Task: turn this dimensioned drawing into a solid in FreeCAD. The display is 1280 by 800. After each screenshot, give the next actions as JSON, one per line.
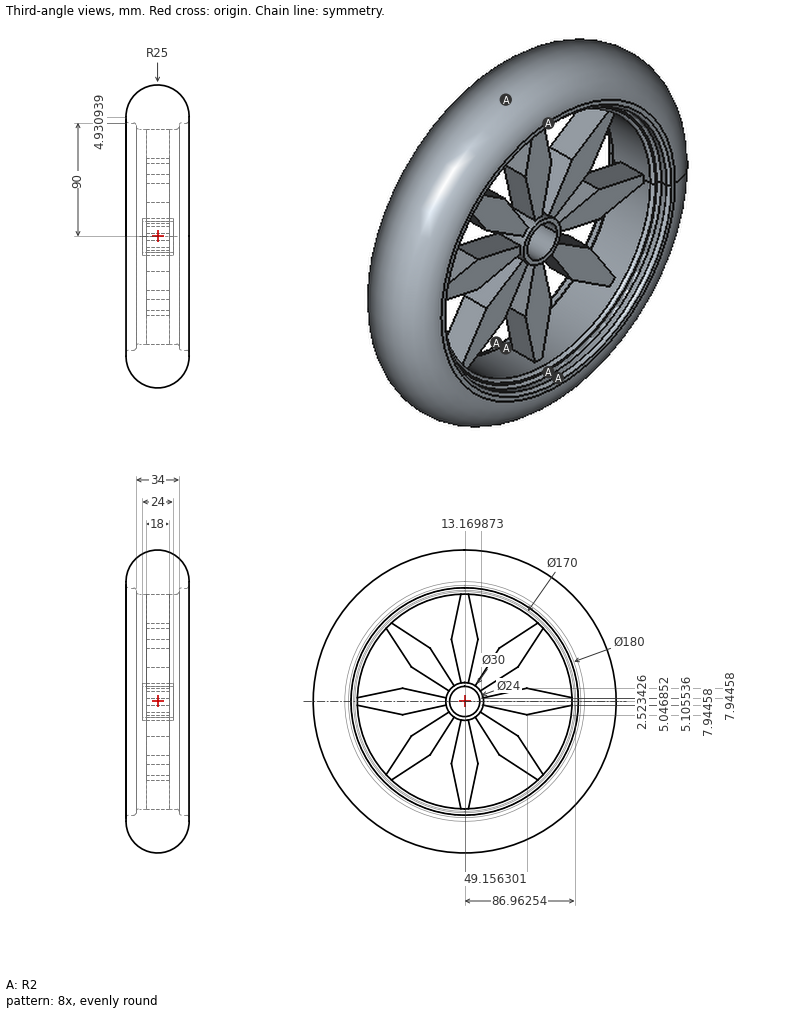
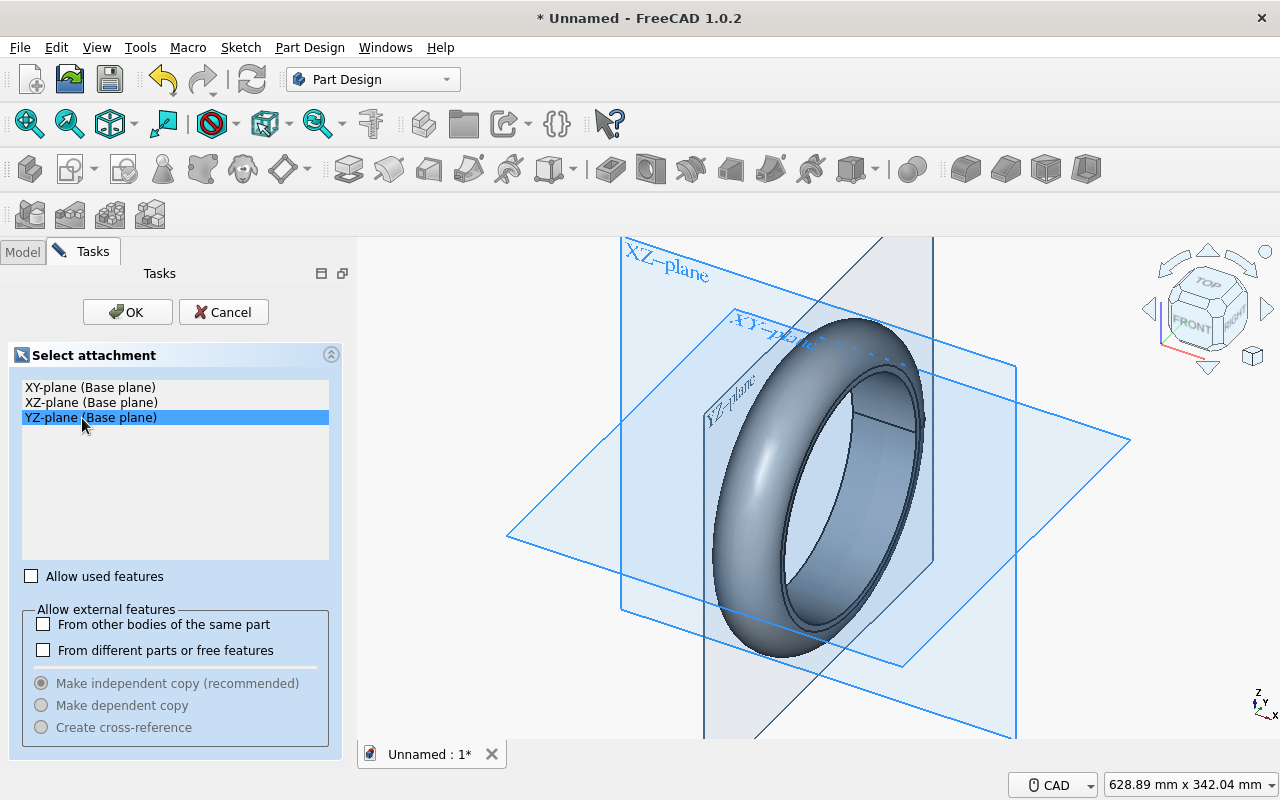
{"action": "left_click", "coordinate": [128, 312]}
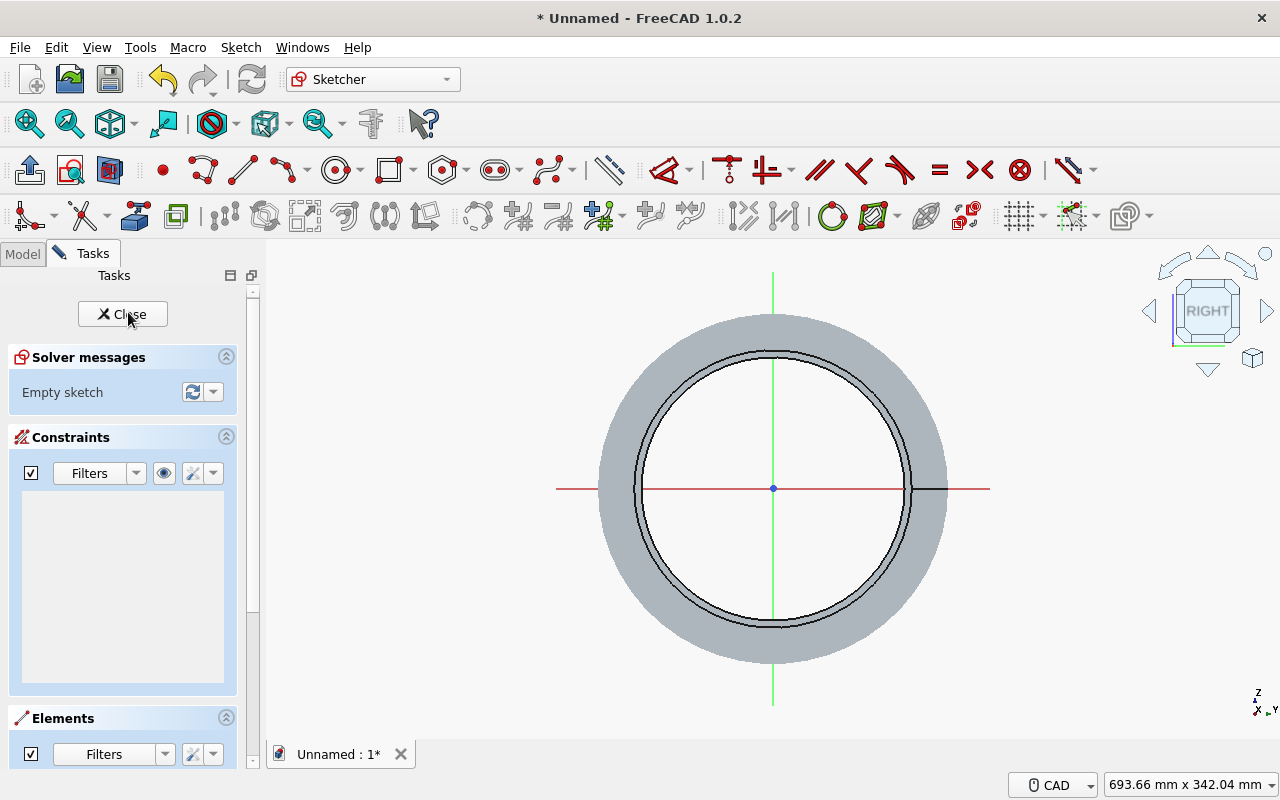
{"action": "left_click", "coordinate": [110, 170]}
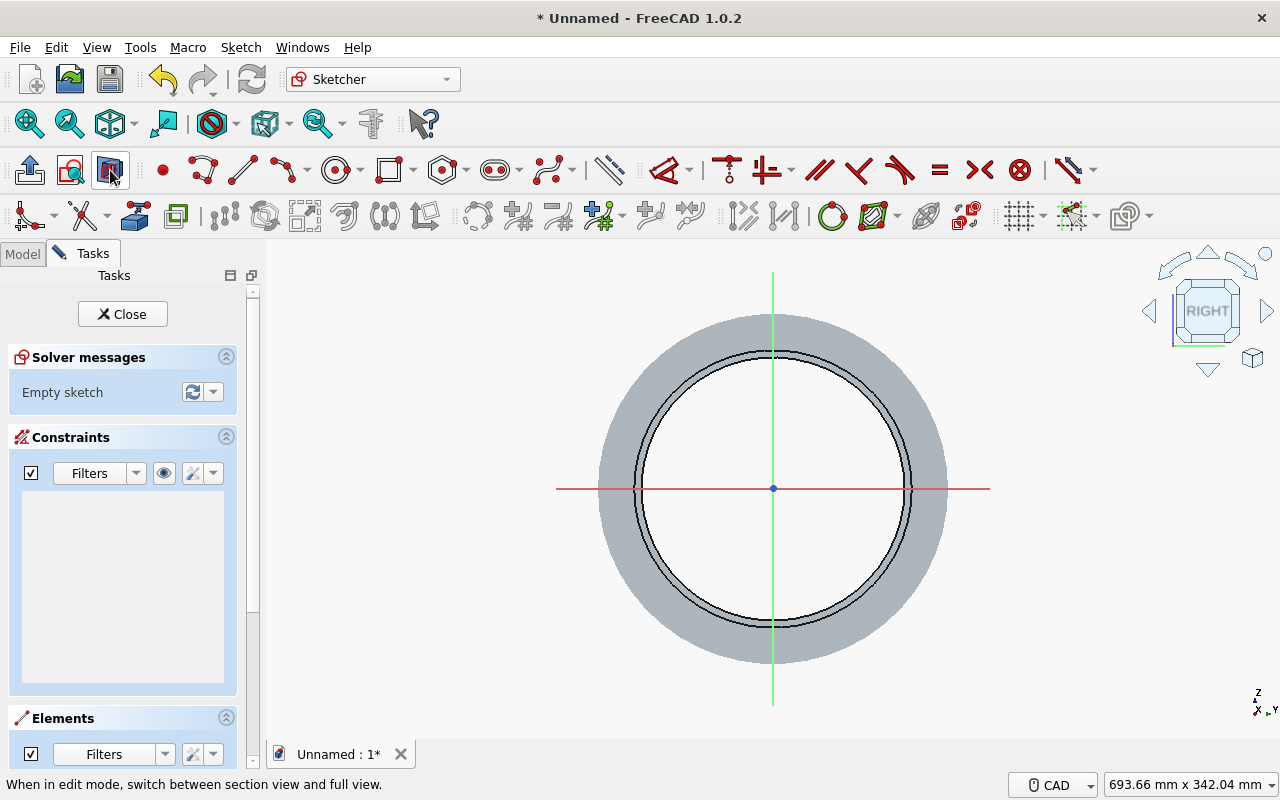
{"action": "key", "text": "g c"}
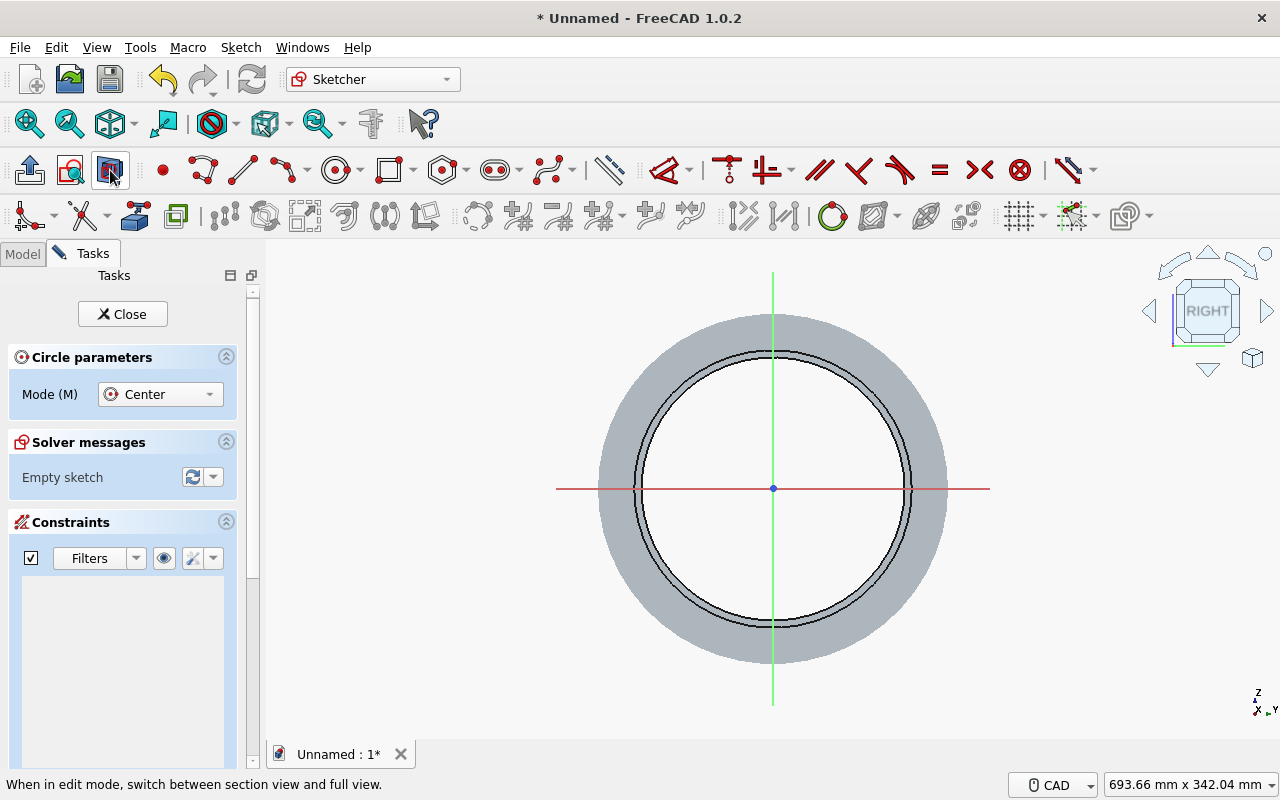
{"action": "left_click", "coordinate": [773, 489]}
{"action": "left_click", "coordinate": [866, 396]}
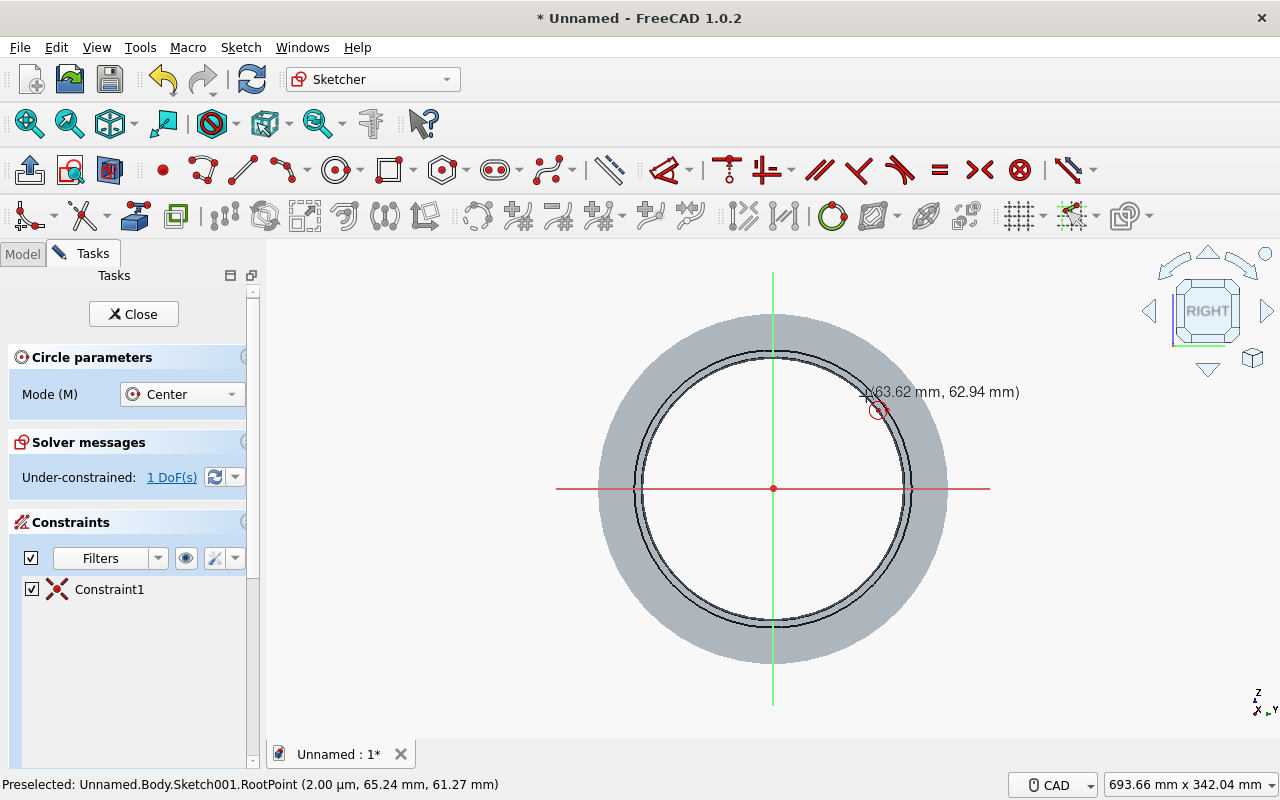
{"action": "left_click", "coordinate": [773, 489]}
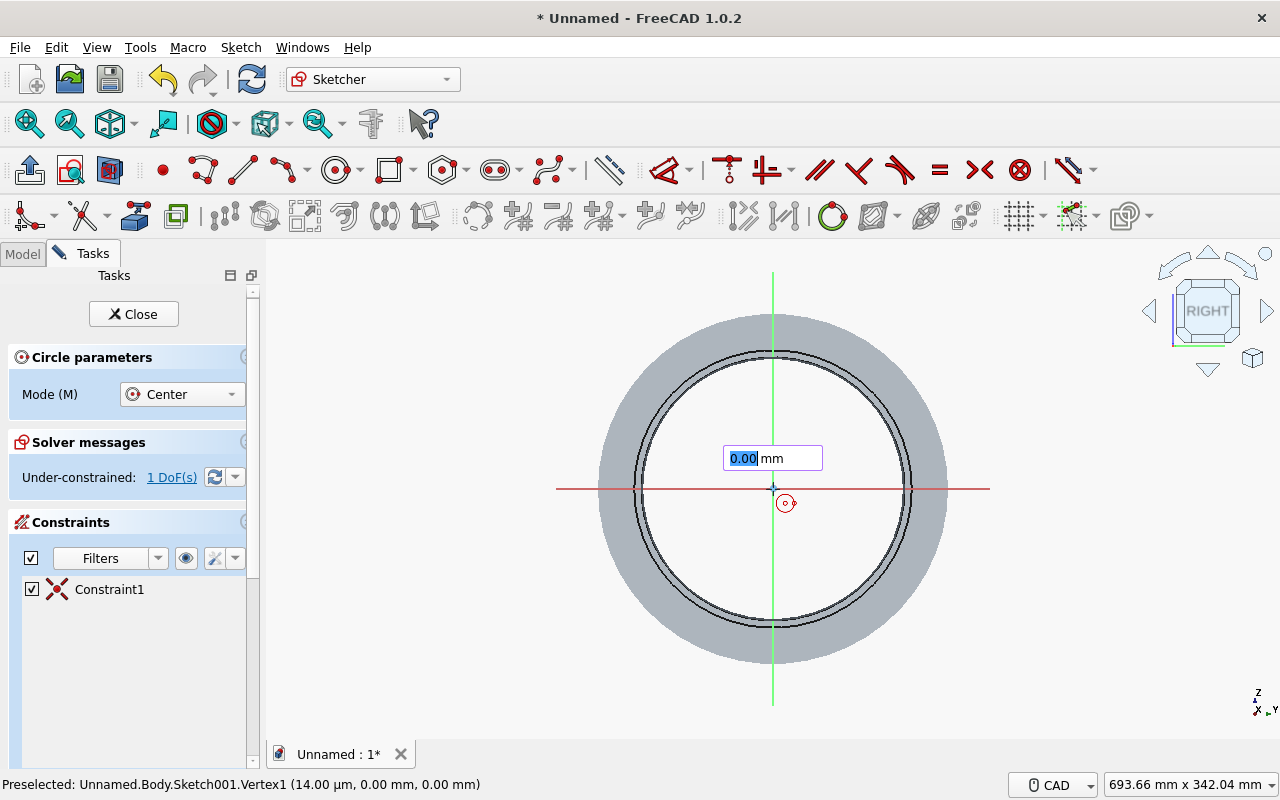
{"action": "scroll", "coordinate": [861, 401], "scroll_direction": "up", "scroll_amount": 4}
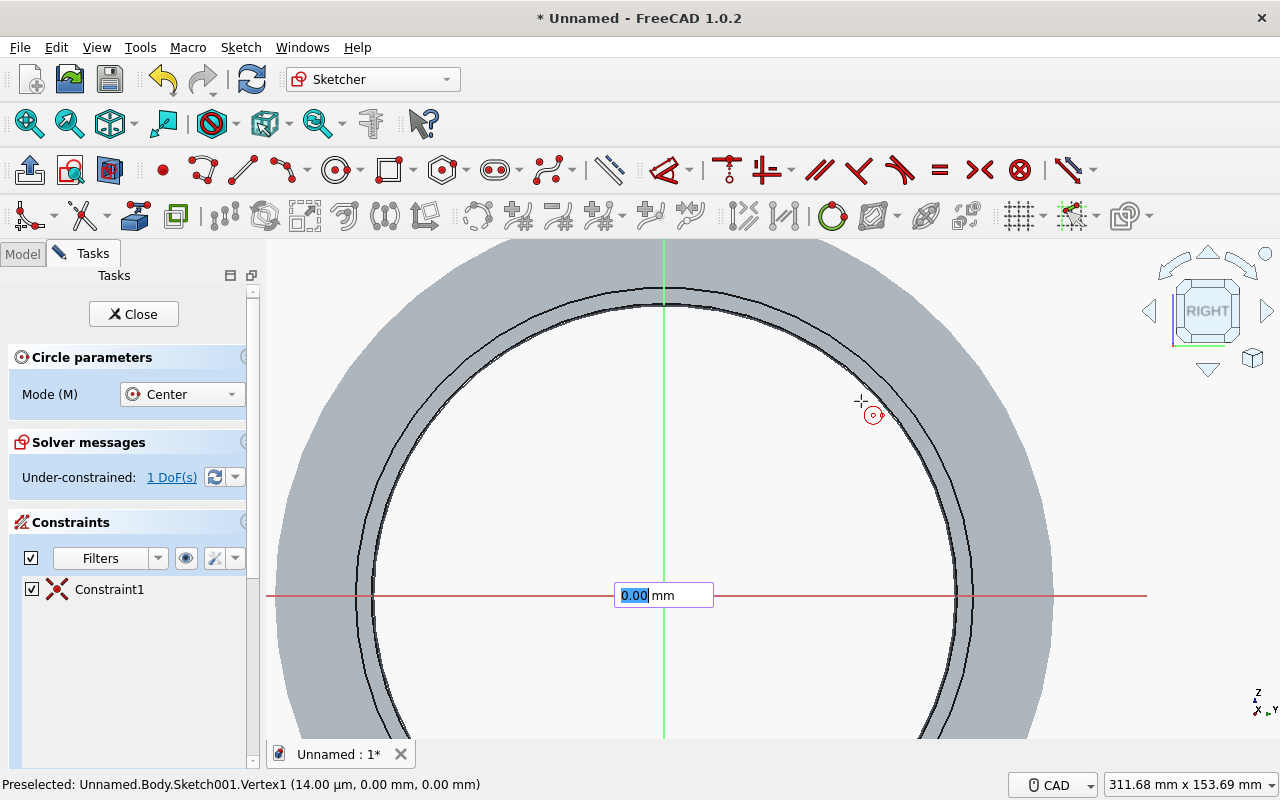
{"action": "left_click", "coordinate": [860, 401]}
{"action": "key", "text": "Escape"}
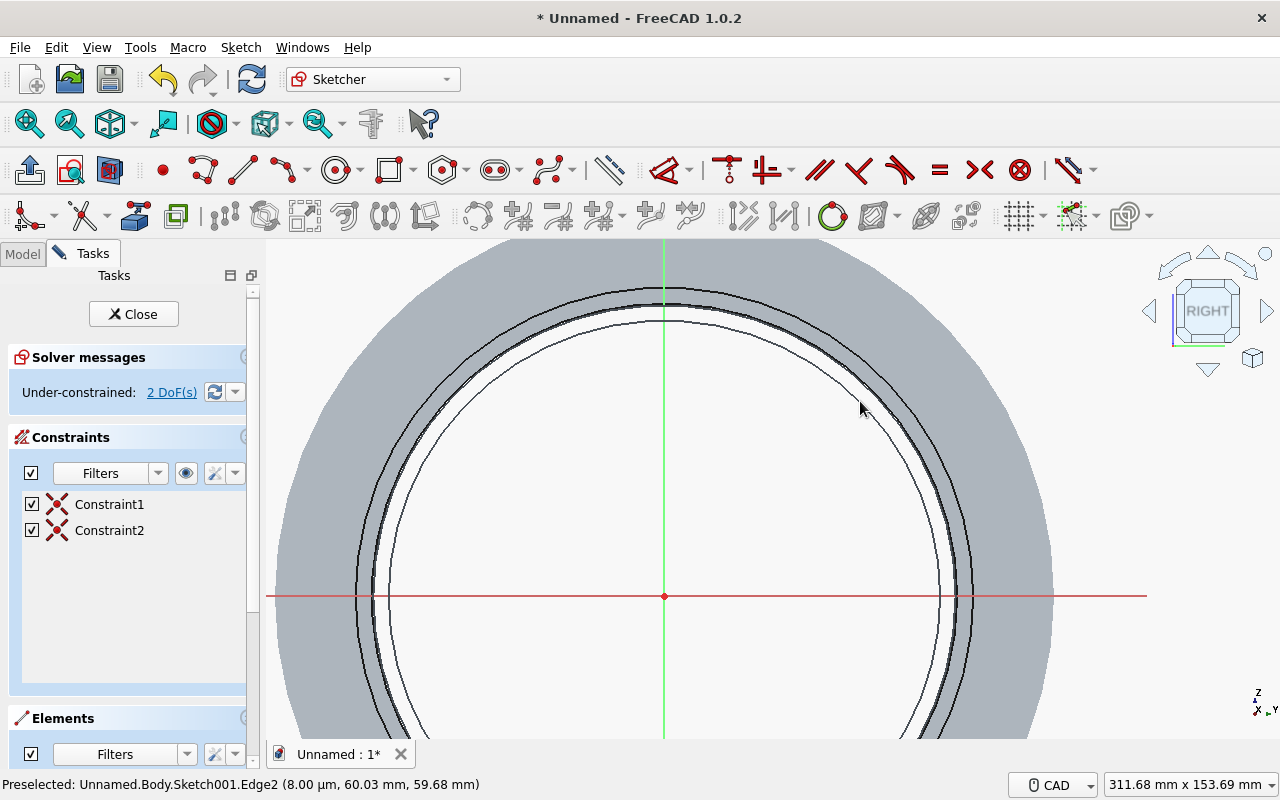
{"action": "left_click", "coordinate": [664, 170]}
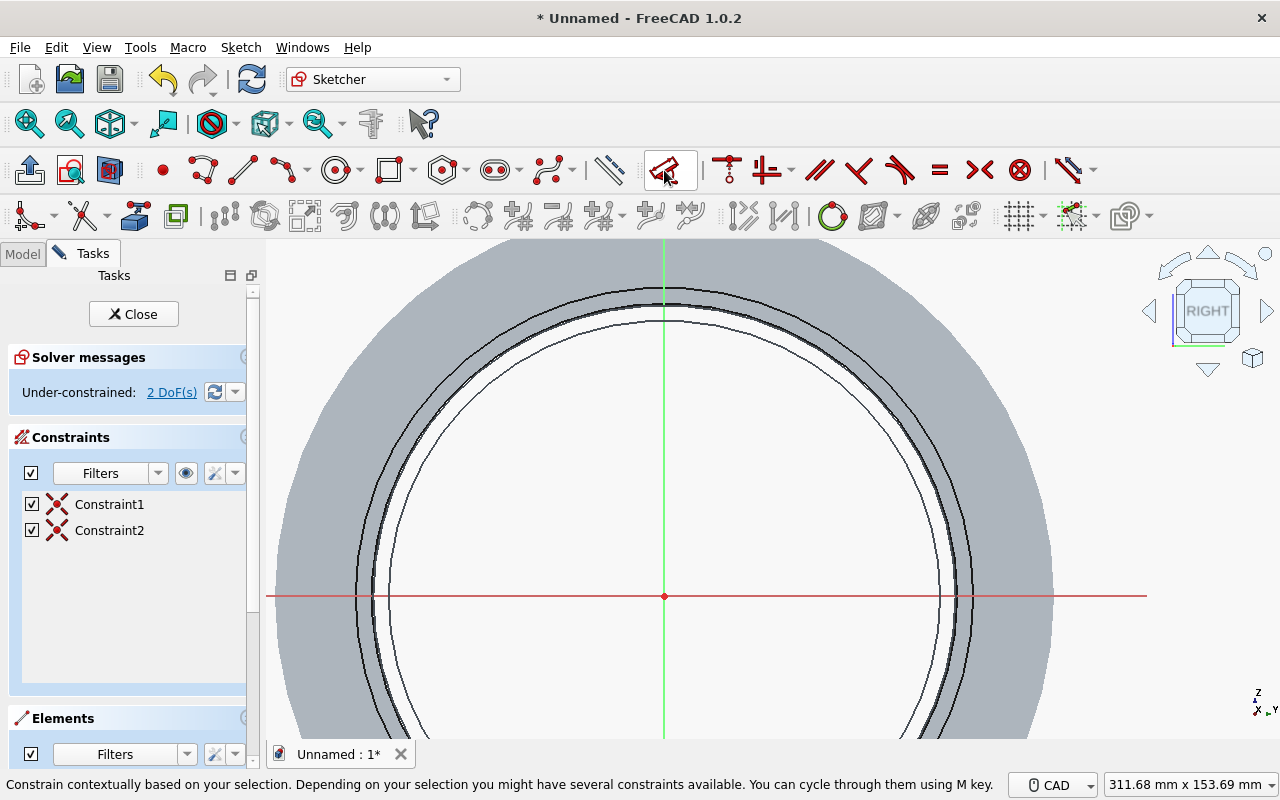
{"action": "left_click", "coordinate": [870, 390]}
{"action": "left_click", "coordinate": [893, 367]}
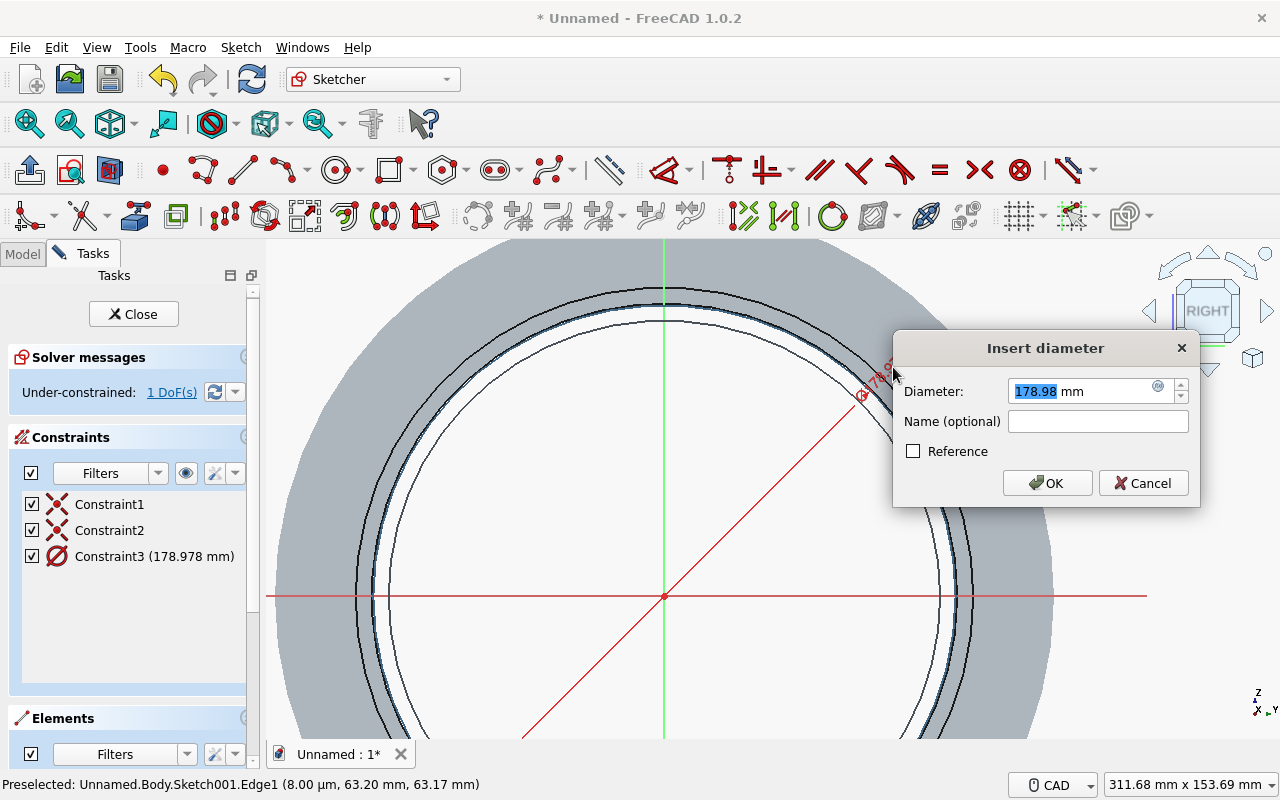
{"action": "type", "text": "180"}
{"action": "key", "text": "Return"}